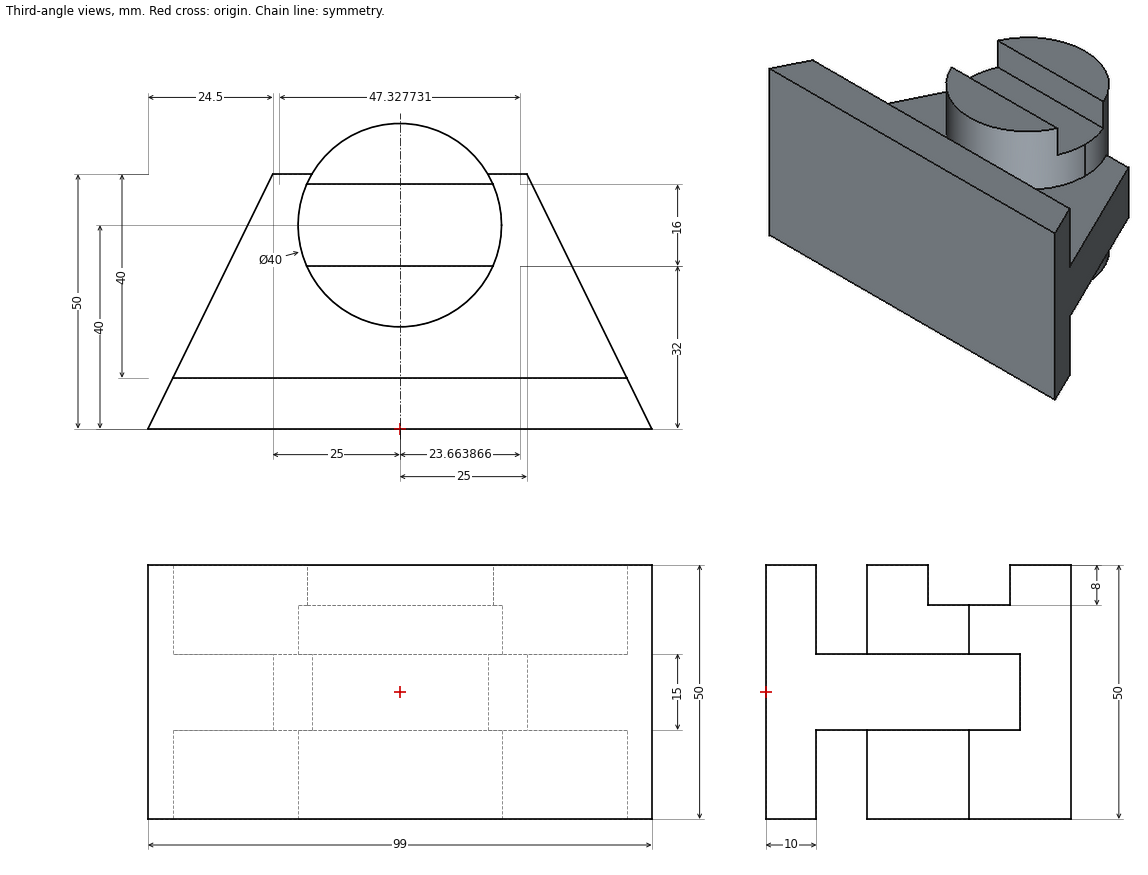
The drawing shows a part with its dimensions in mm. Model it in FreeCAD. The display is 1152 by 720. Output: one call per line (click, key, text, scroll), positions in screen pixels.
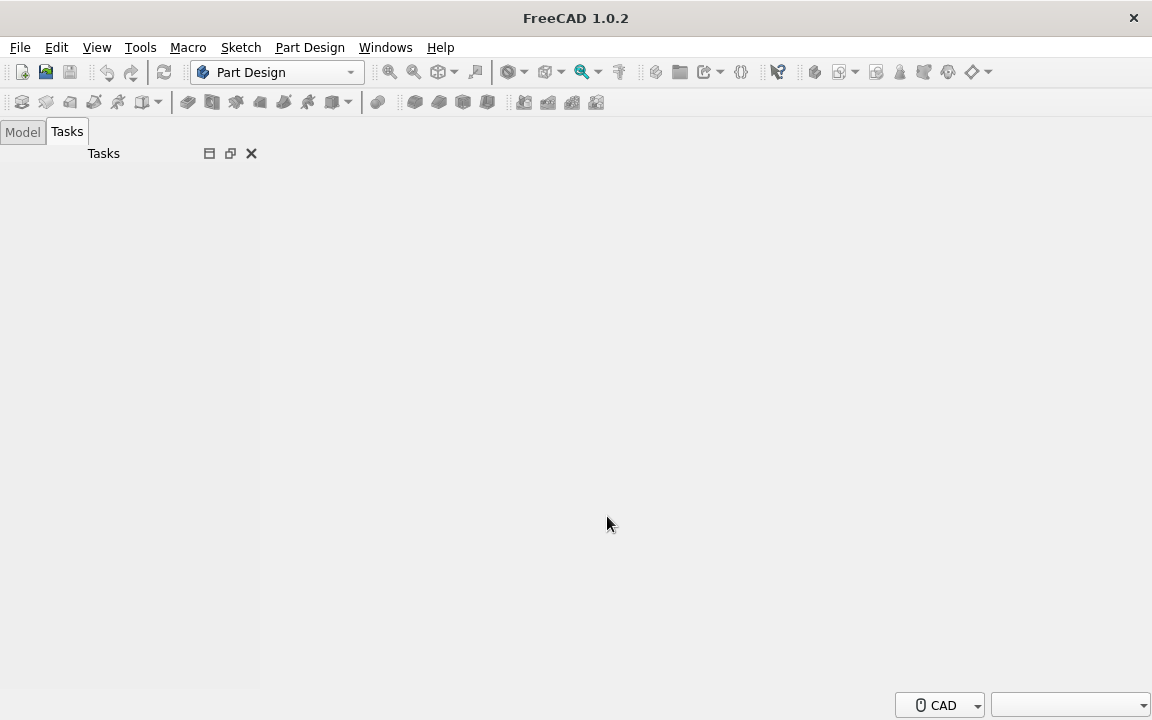
key(ctrl+n)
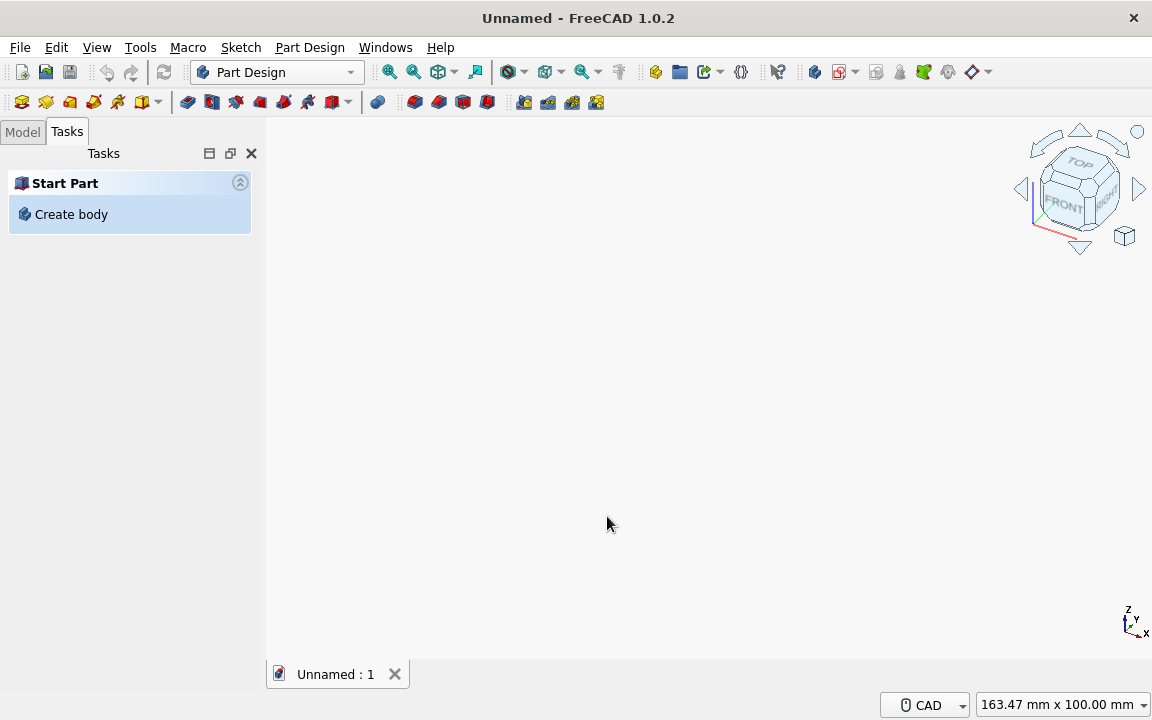
click(840, 72)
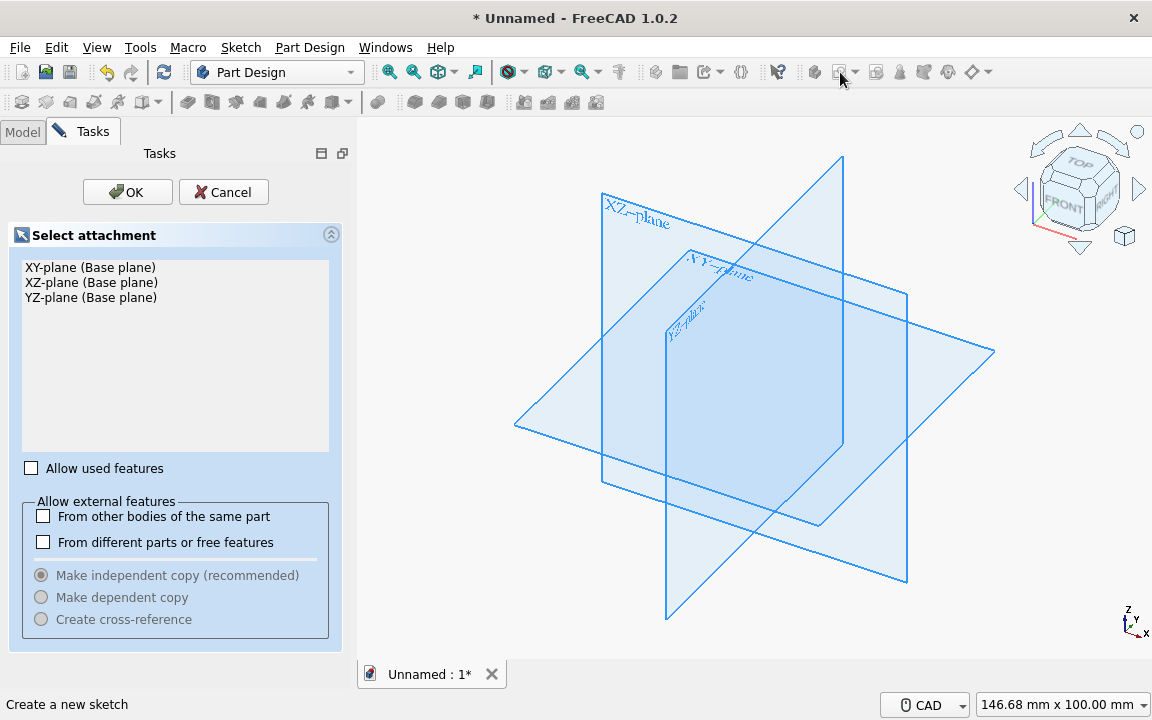
click(82, 282)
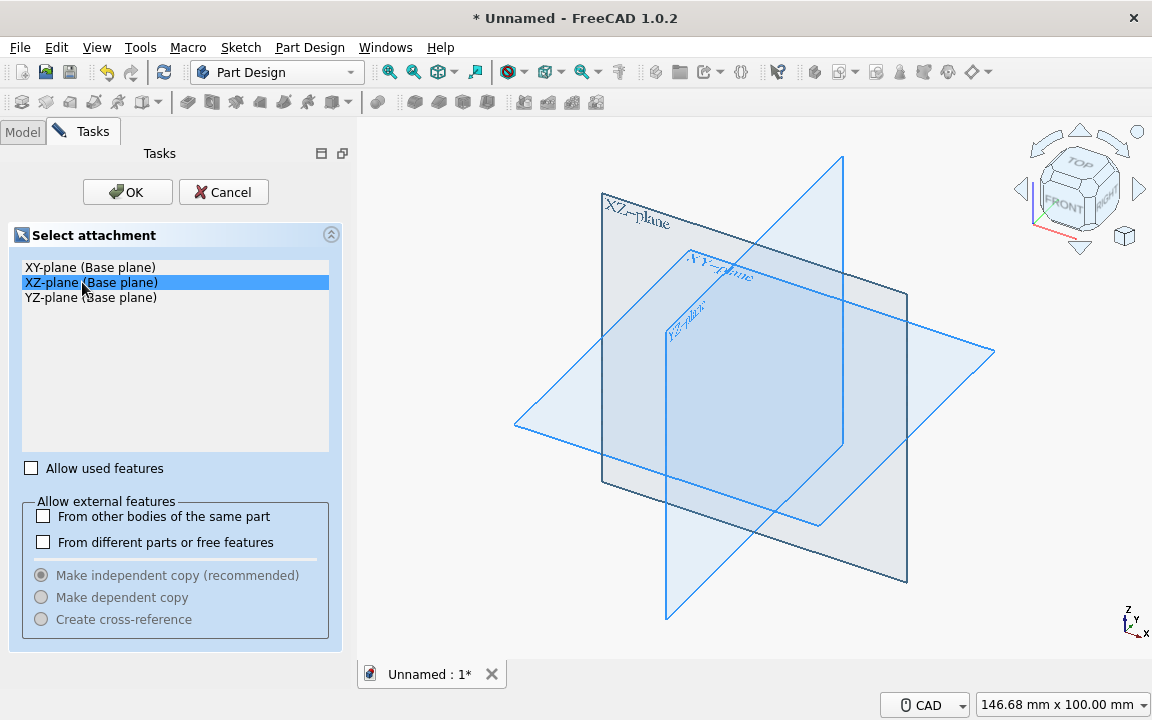
click(128, 192)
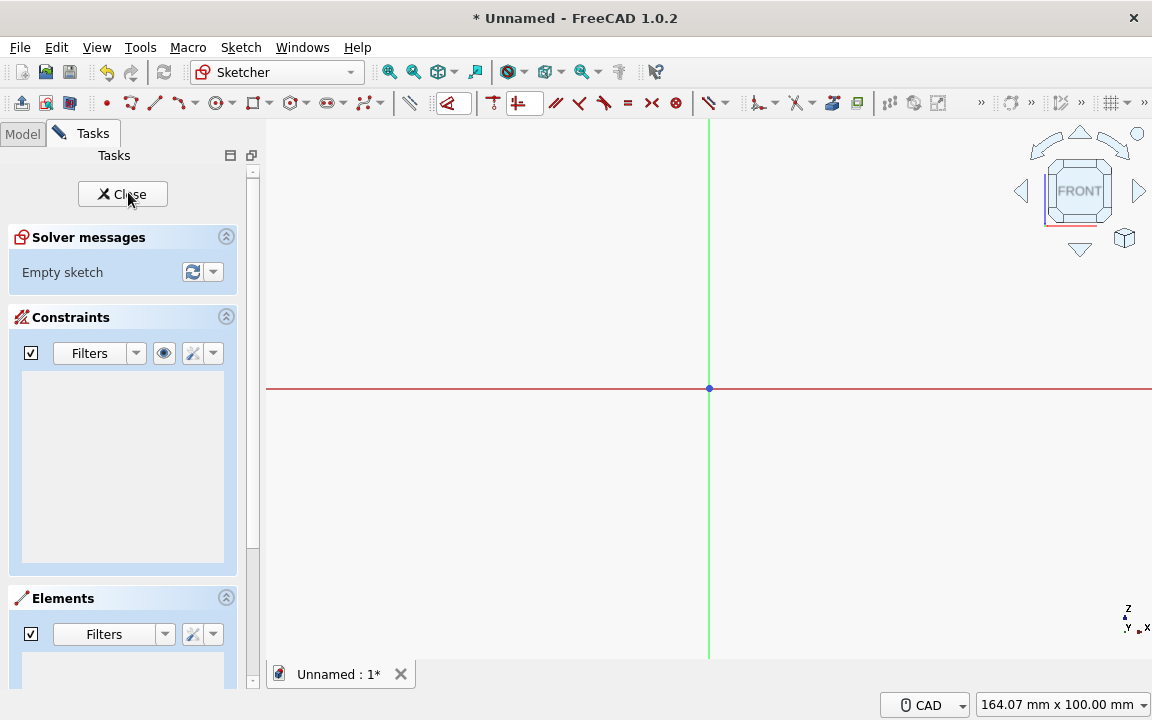
scroll(331, 389, down, 1)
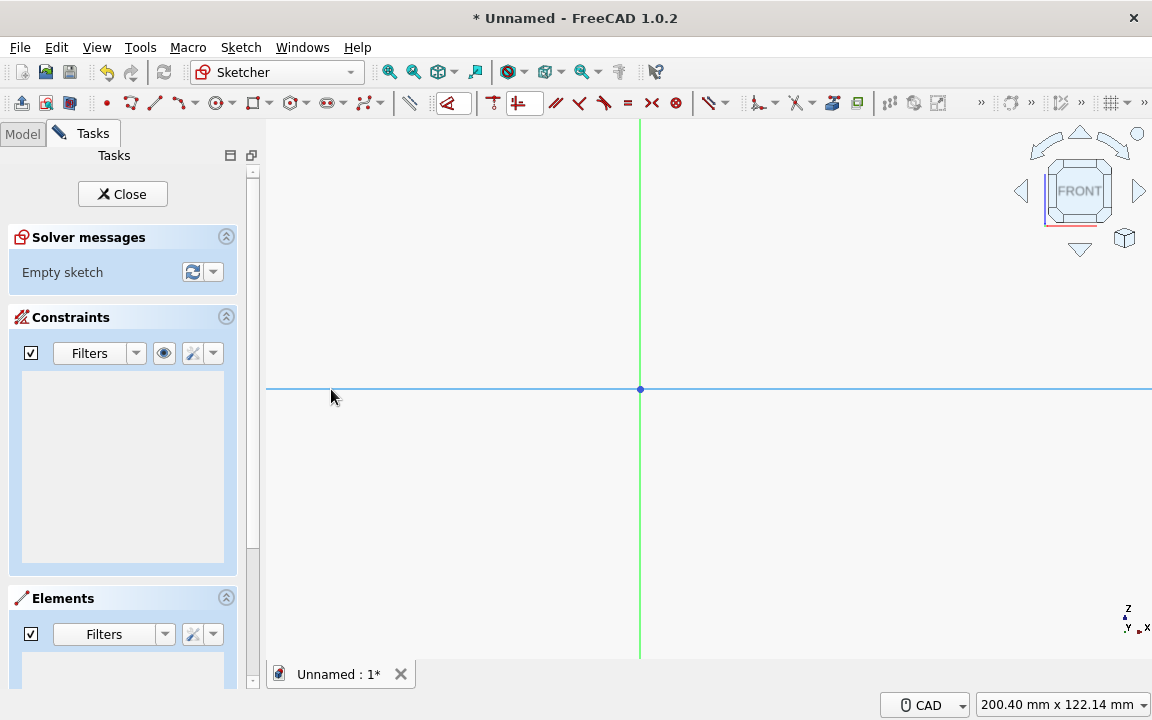
key(g)
key(v)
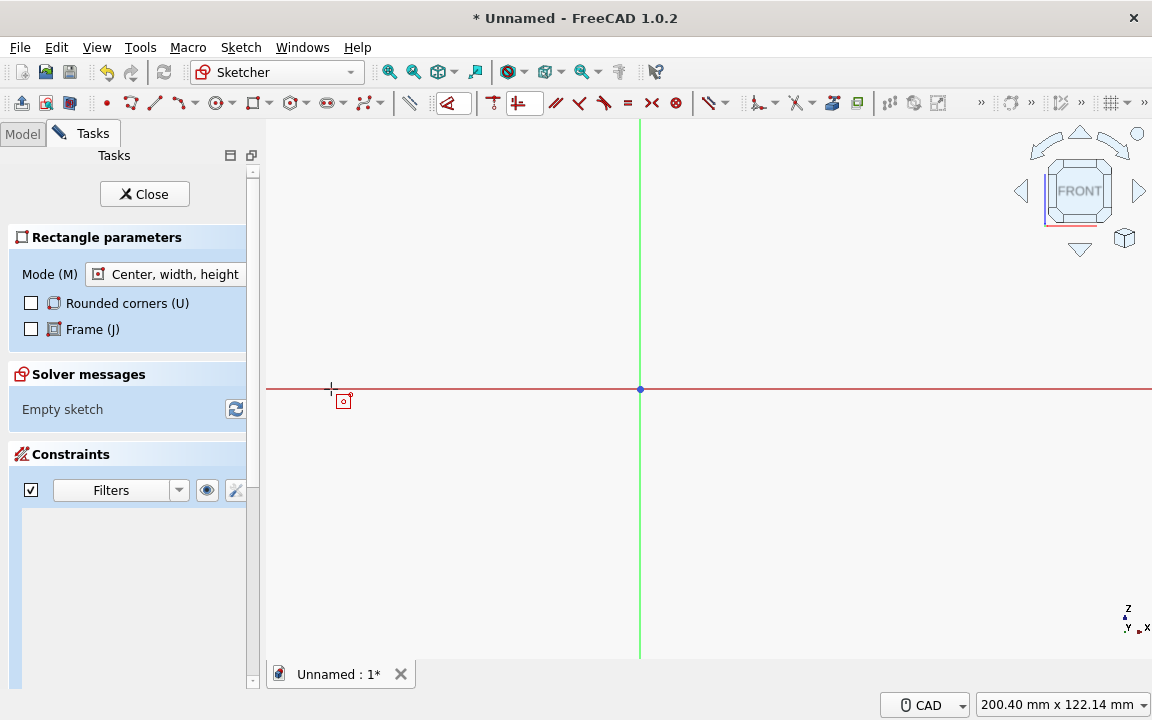
click(640, 389)
click(859, 279)
key(Escape)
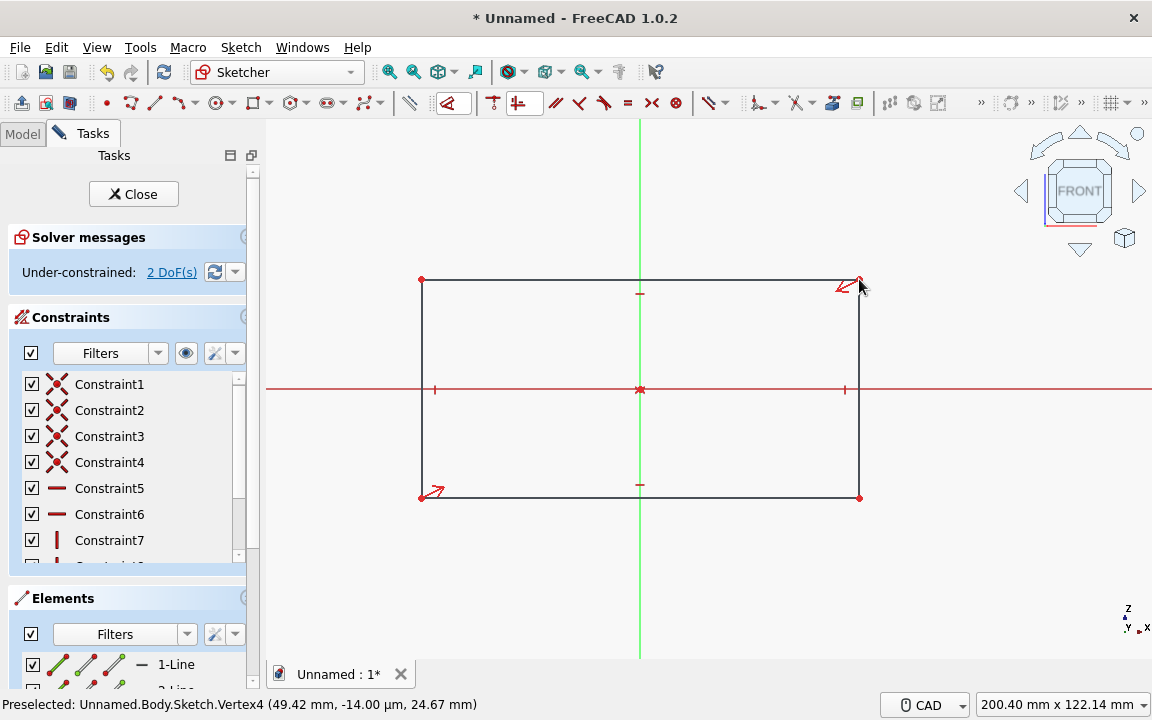
key(d)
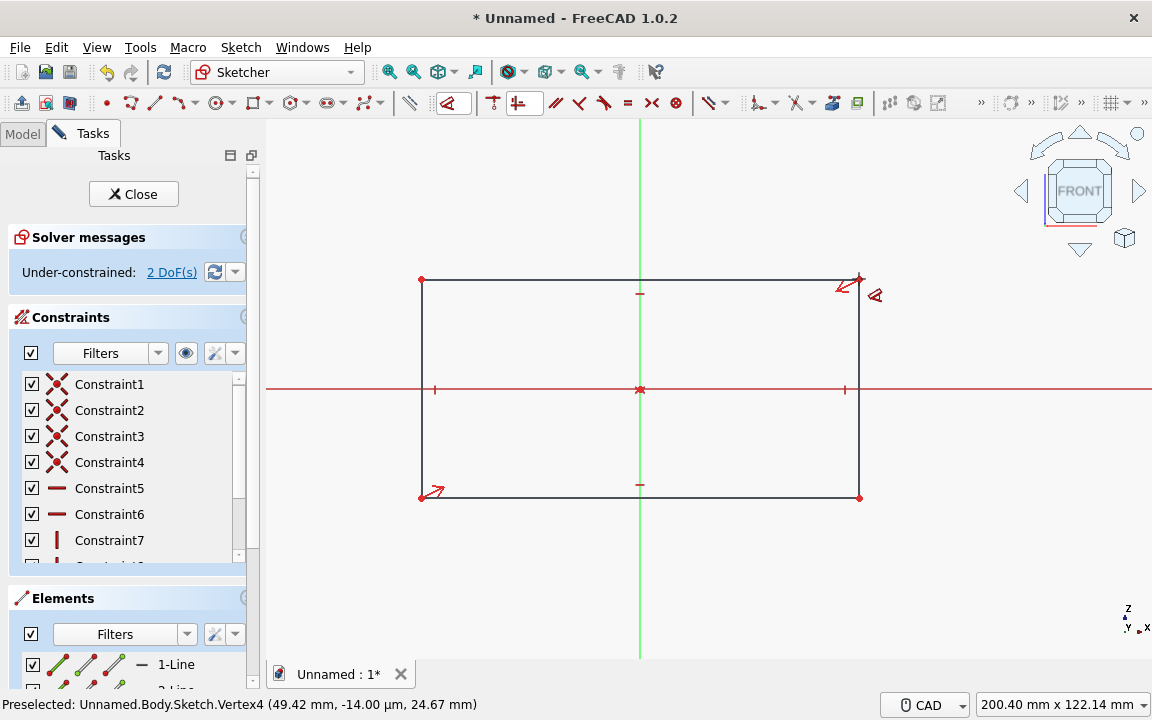
click(553, 498)
click(540, 532)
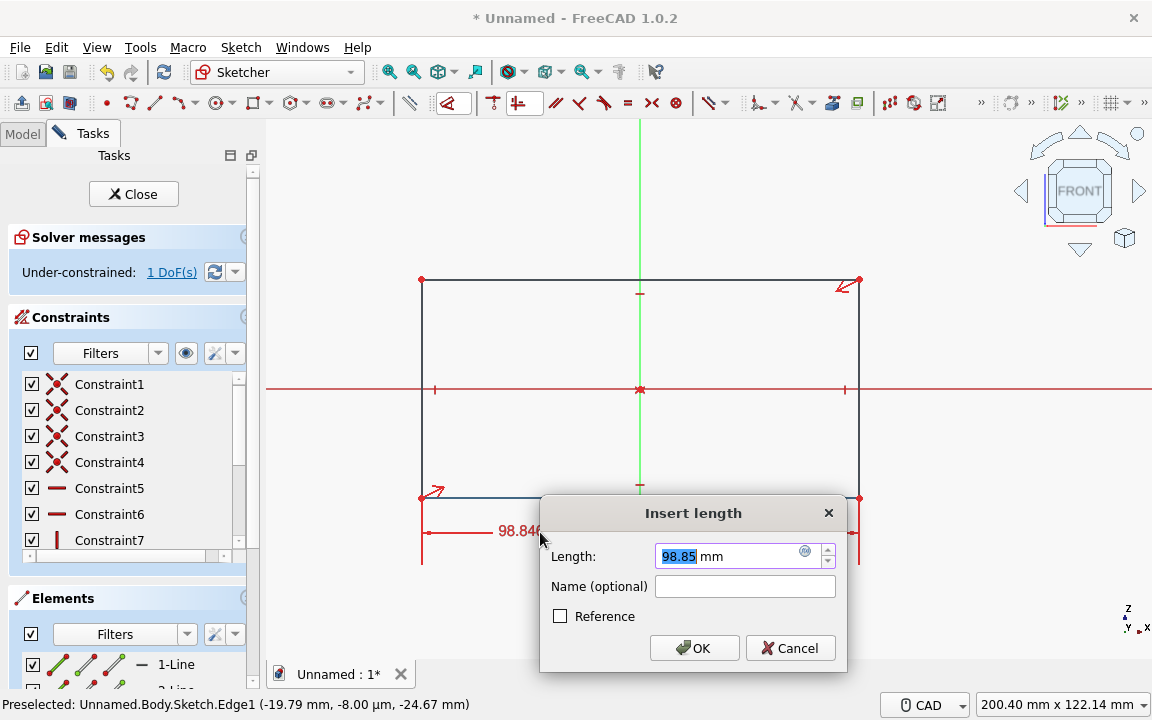
text(99)
key(Return)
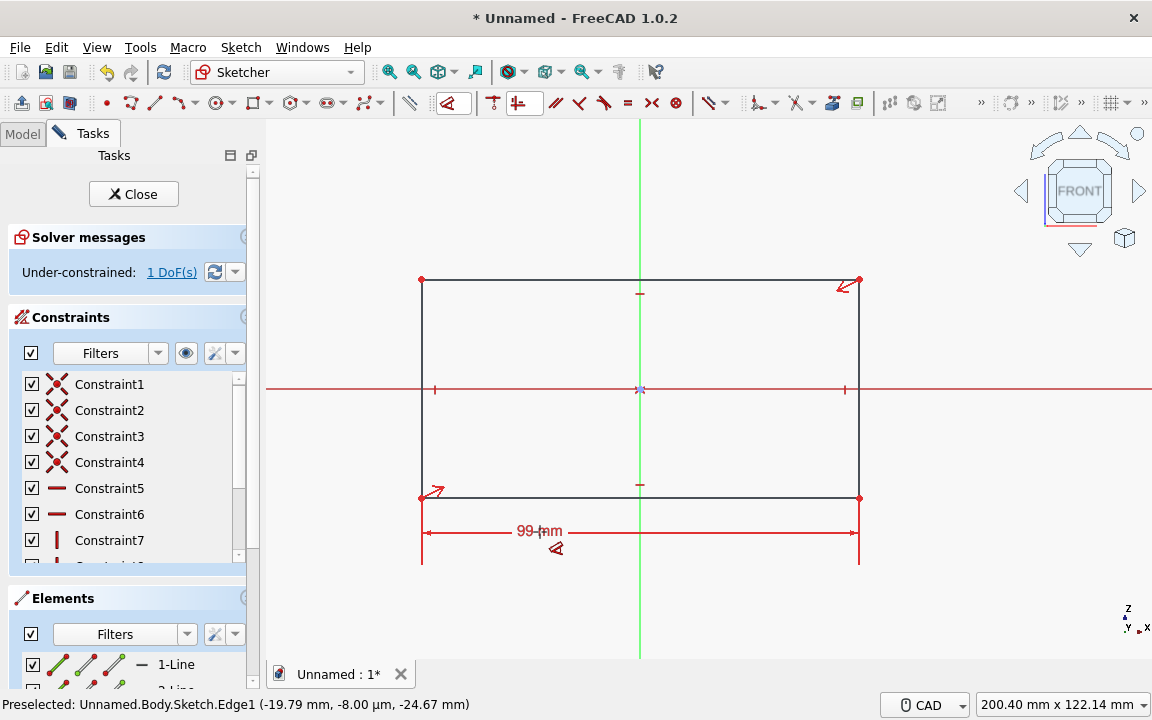
click(859, 433)
click(893, 339)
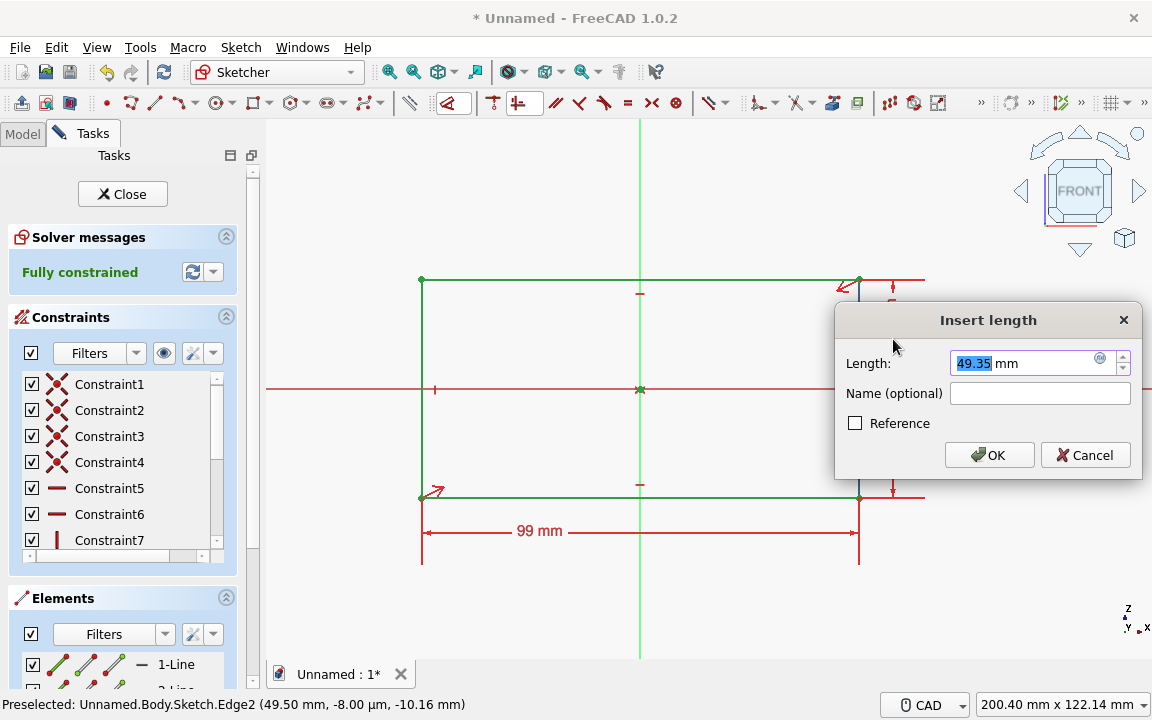
text(50)
key(Return)
key(Escape)